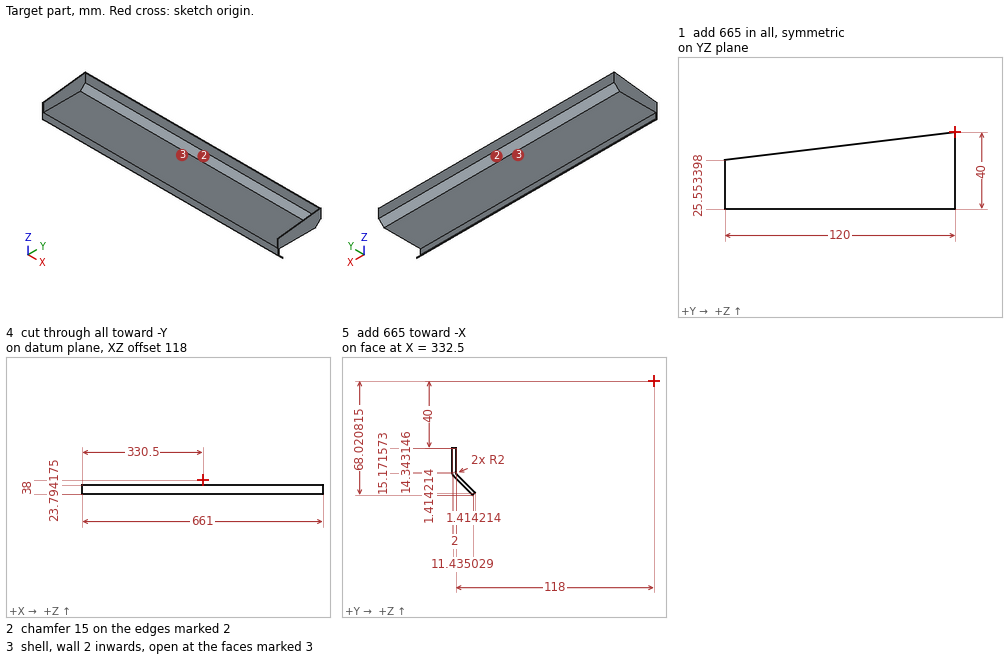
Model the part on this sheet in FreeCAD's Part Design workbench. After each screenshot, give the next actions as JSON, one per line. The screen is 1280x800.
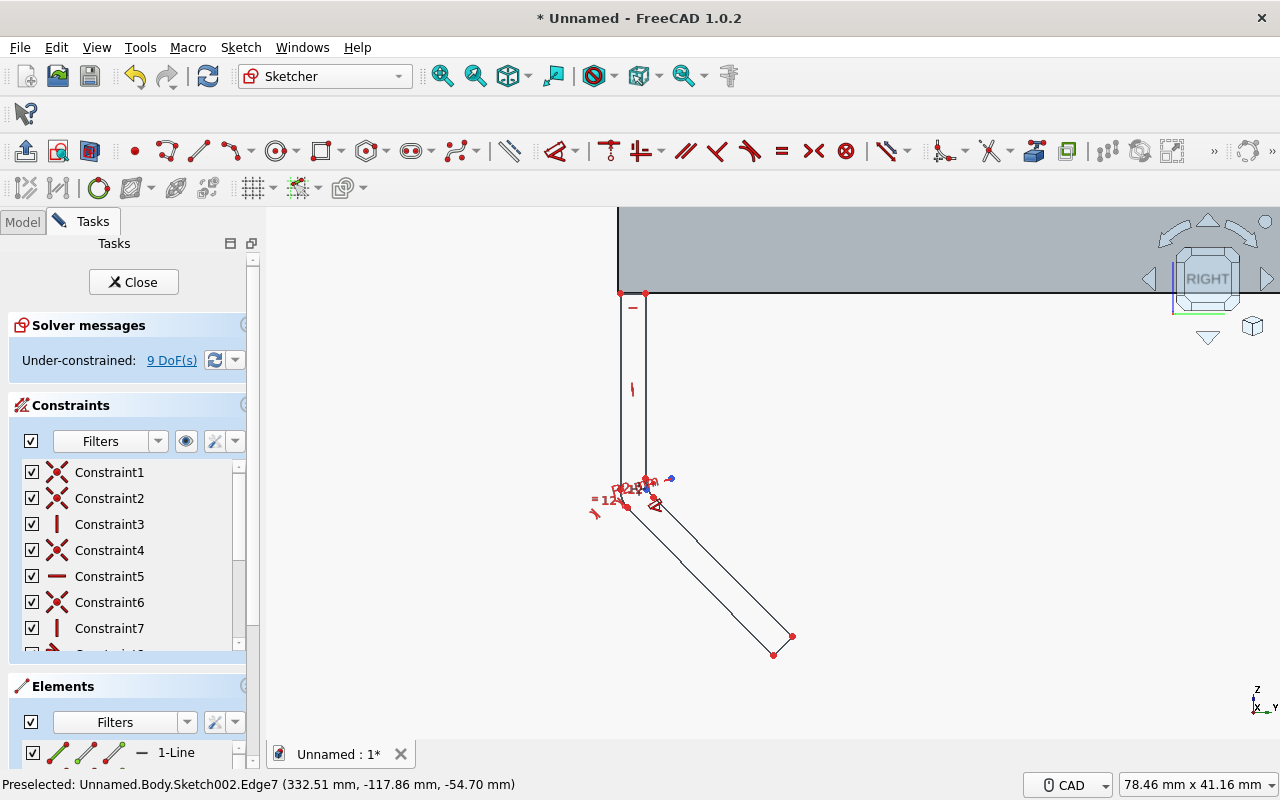
{"action": "scroll", "coordinate": [638, 294], "scroll_direction": "up", "scroll_amount": 3}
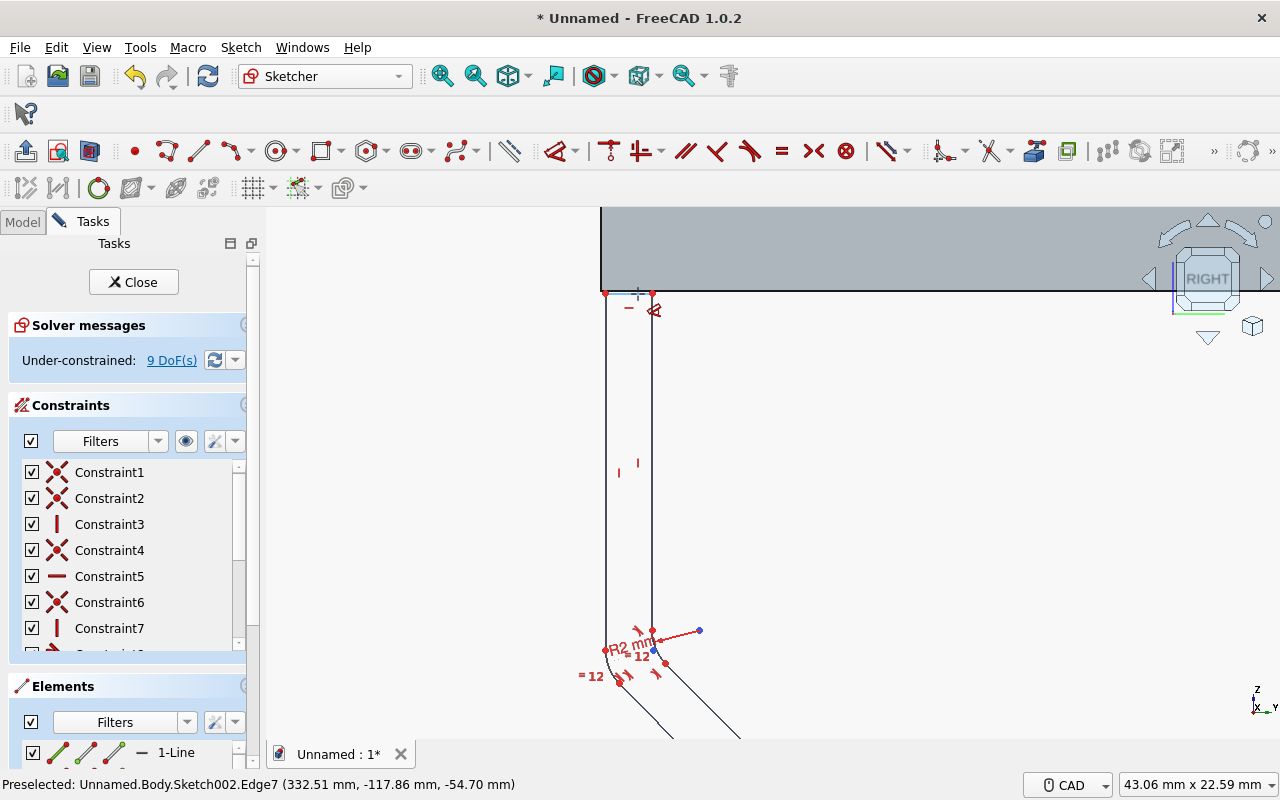
{"action": "left_click", "coordinate": [638, 294]}
{"action": "left_click", "coordinate": [629, 260]}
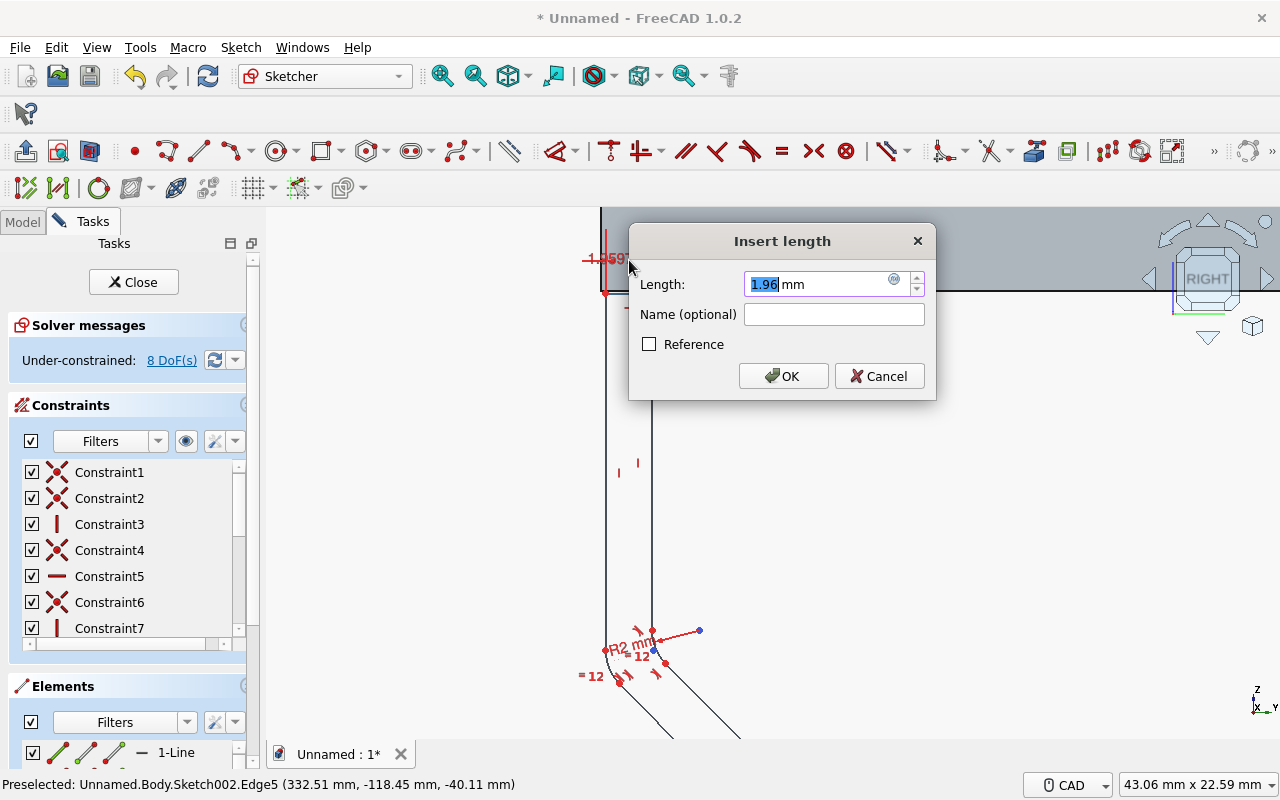
{"action": "type", "text": "2"}
{"action": "key", "text": "Return"}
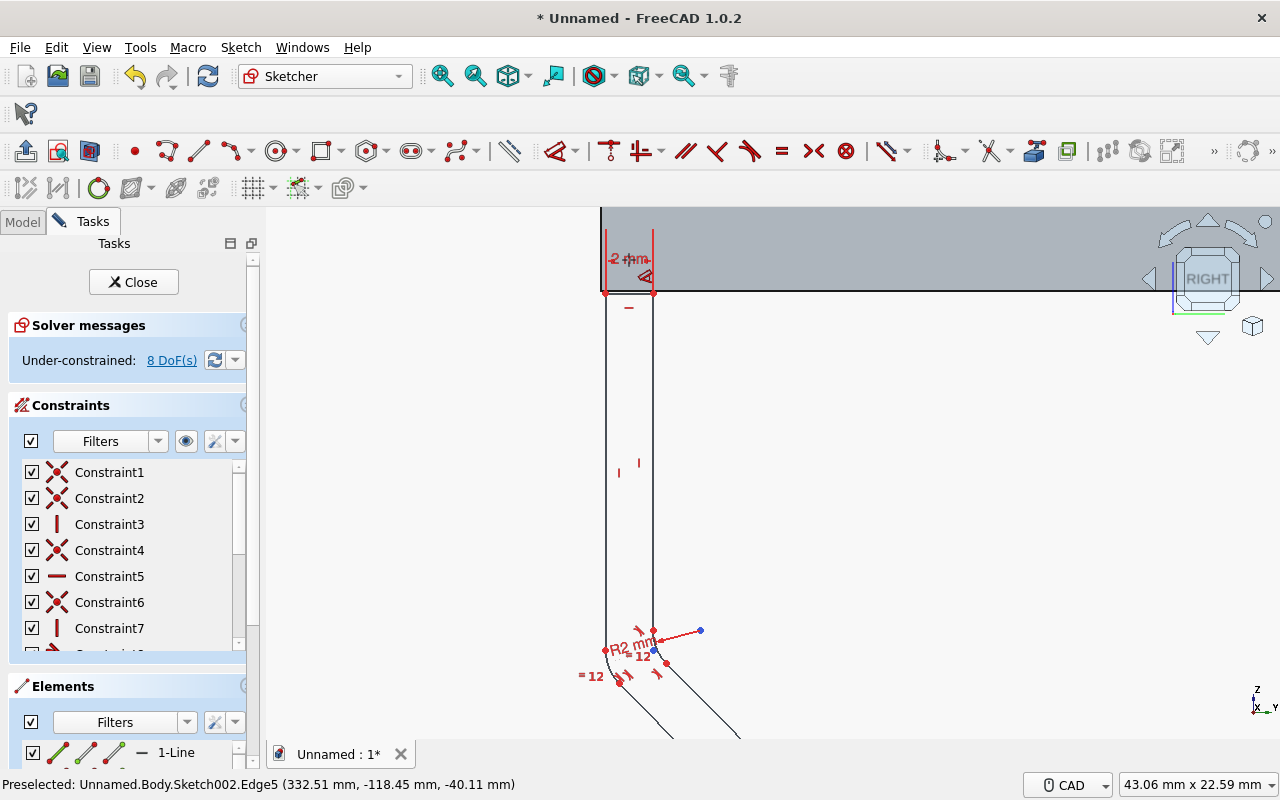
{"action": "left_click", "coordinate": [653, 294]}
{"action": "left_click", "coordinate": [595, 285]}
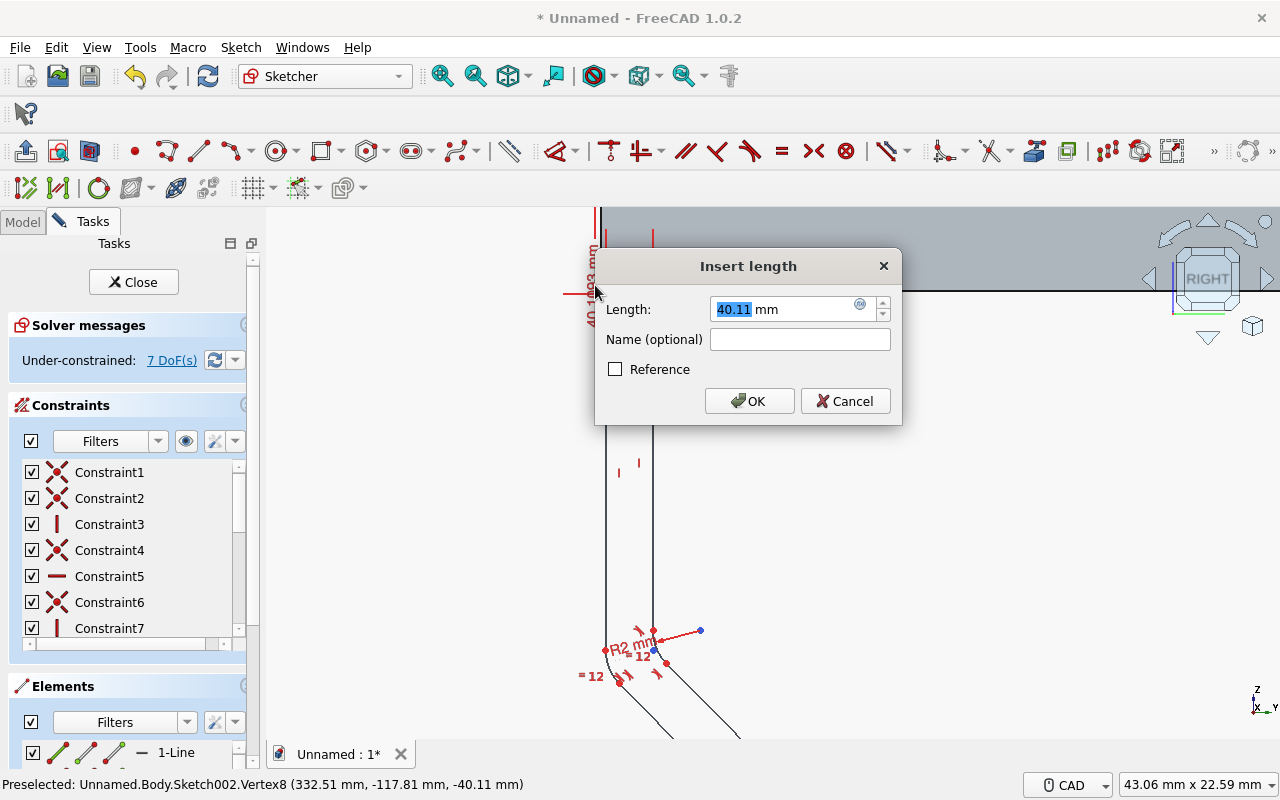
{"action": "type", "text": "40"}
{"action": "key", "text": "Return"}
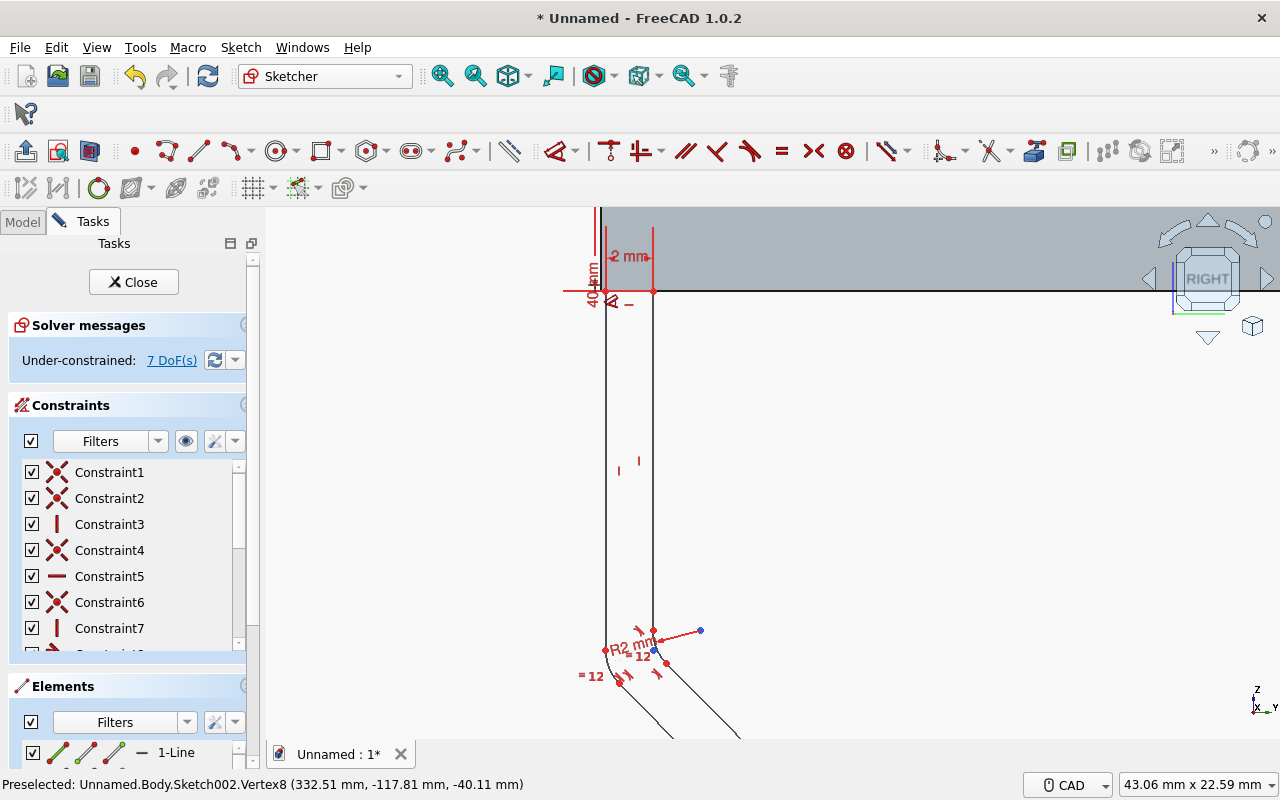
{"action": "left_click", "coordinate": [653, 631]}
{"action": "left_click", "coordinate": [884, 665]}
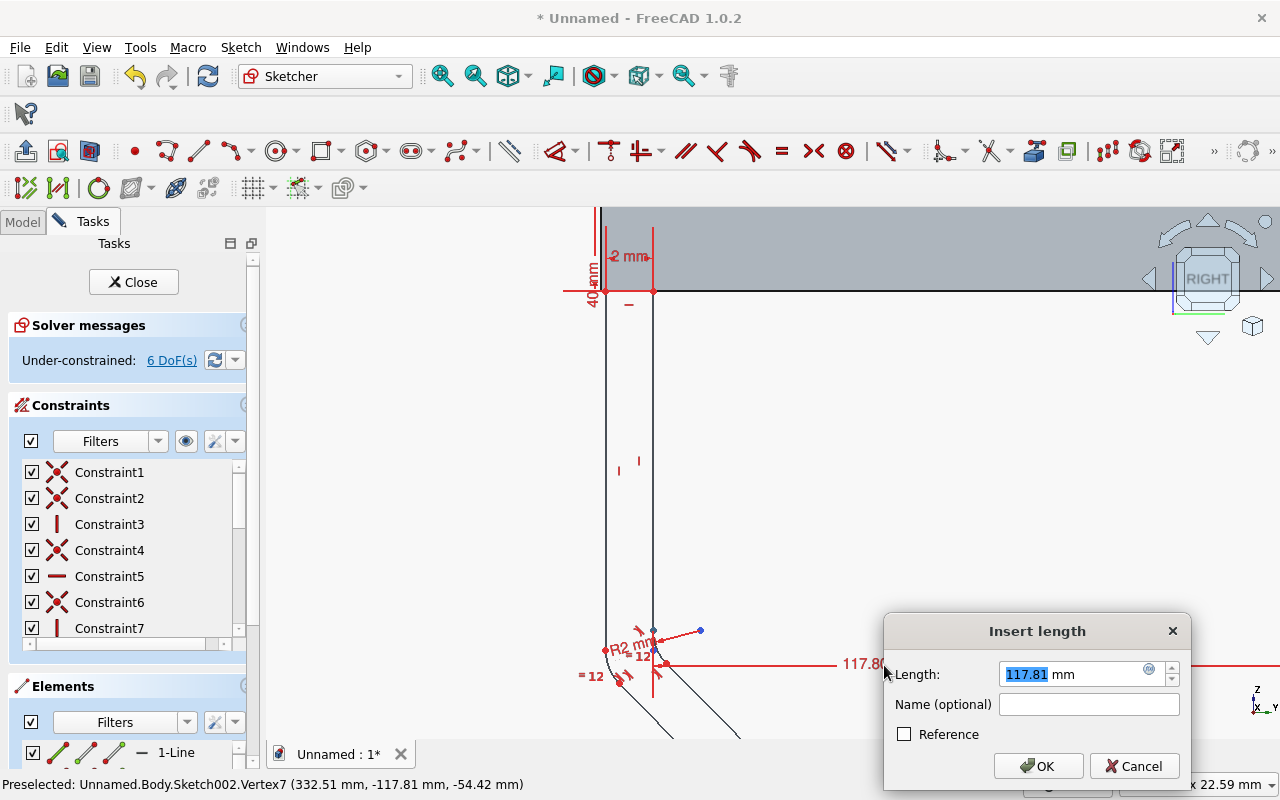
{"action": "type", "text": "118"}
{"action": "key", "text": "Return"}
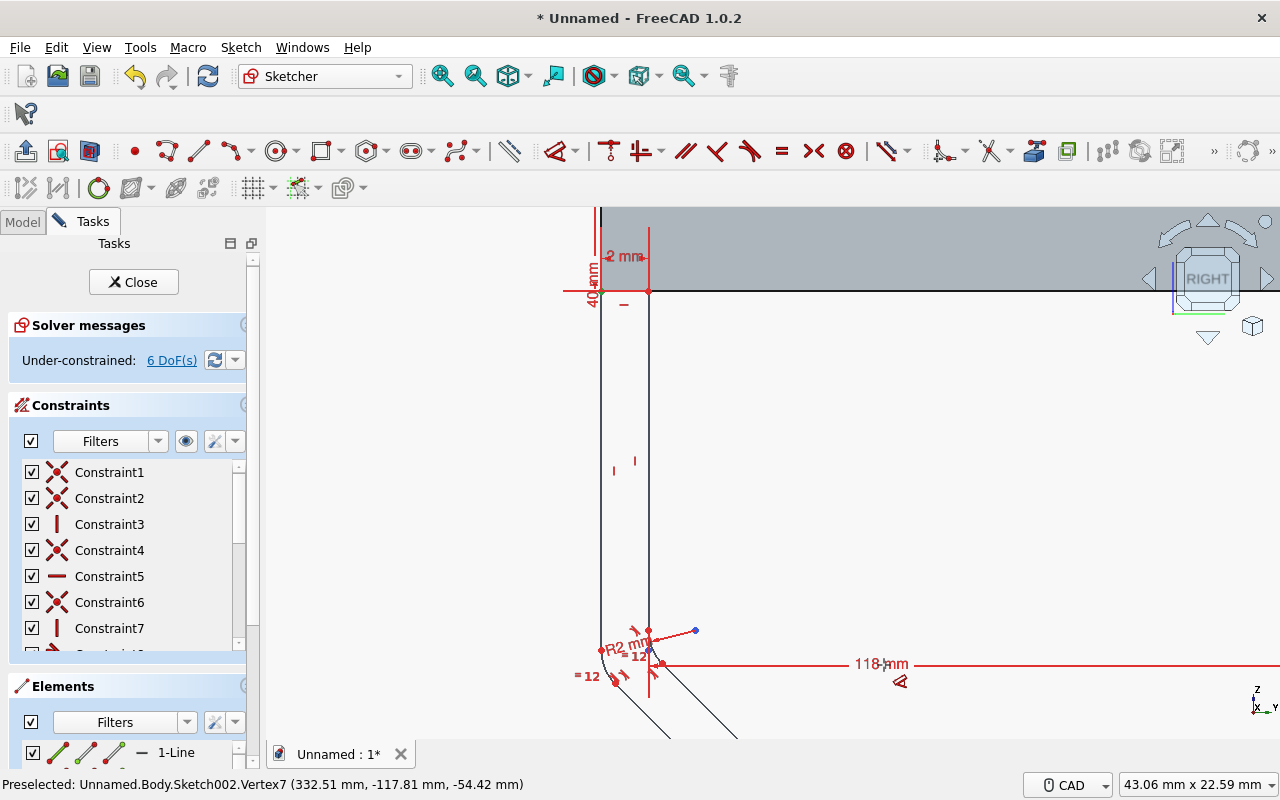
{"action": "left_click", "coordinate": [649, 529]}
{"action": "left_click", "coordinate": [615, 461]}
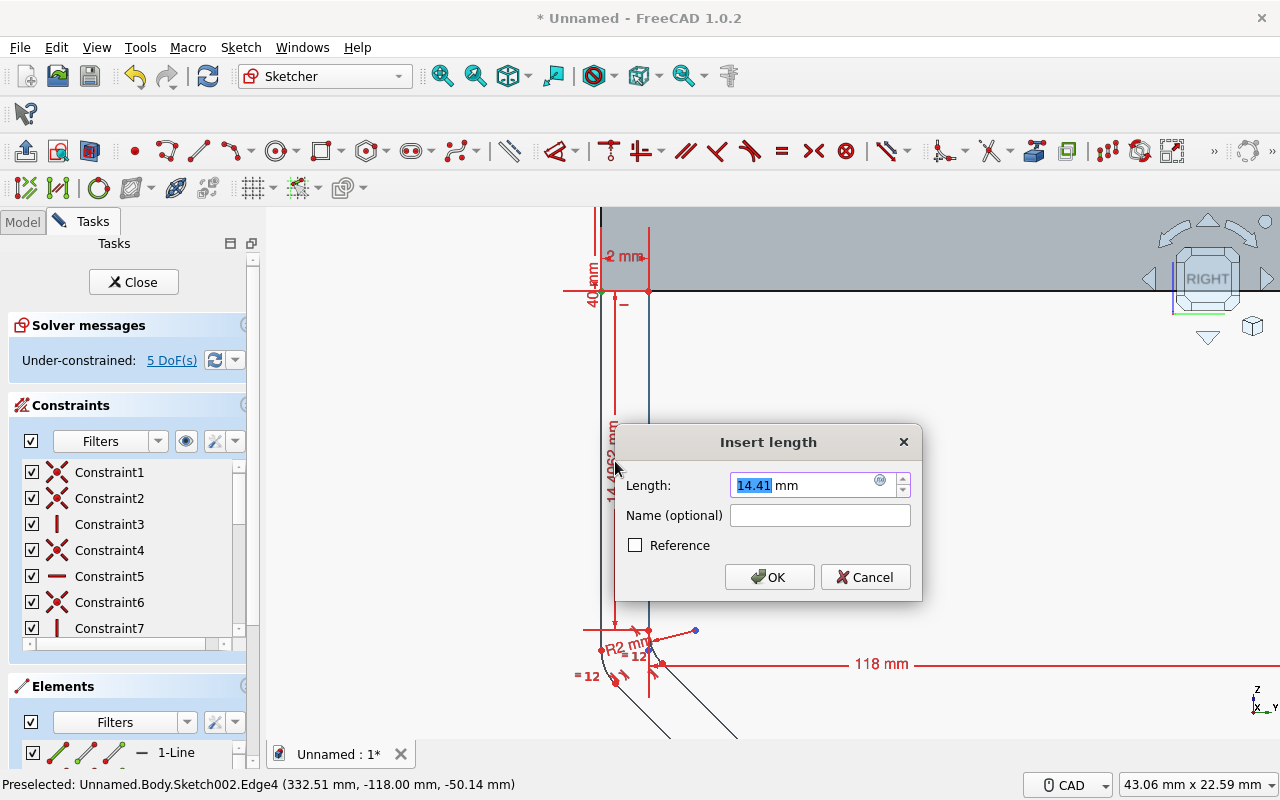
{"action": "type", "text": "14.343146"}
{"action": "key", "text": "Return"}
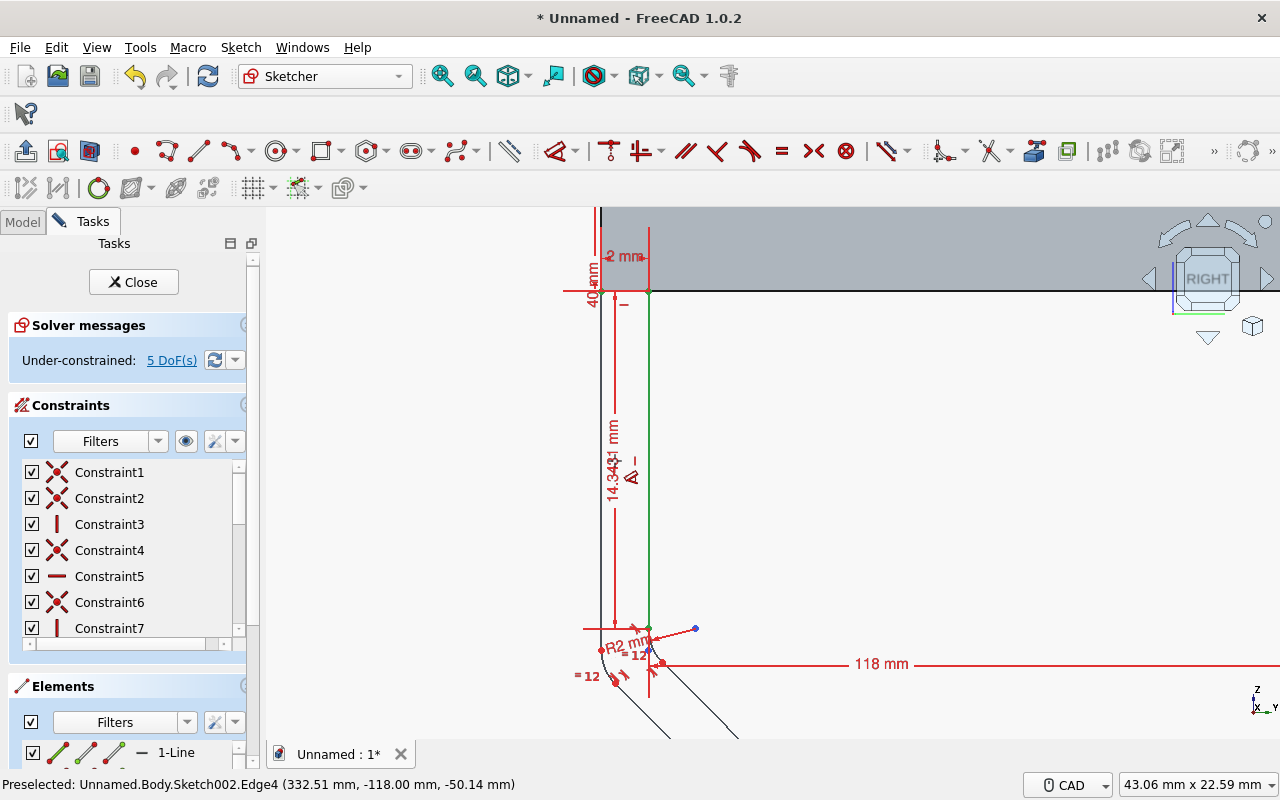
{"action": "left_click", "coordinate": [601, 399]}
{"action": "left_click", "coordinate": [567, 388]}